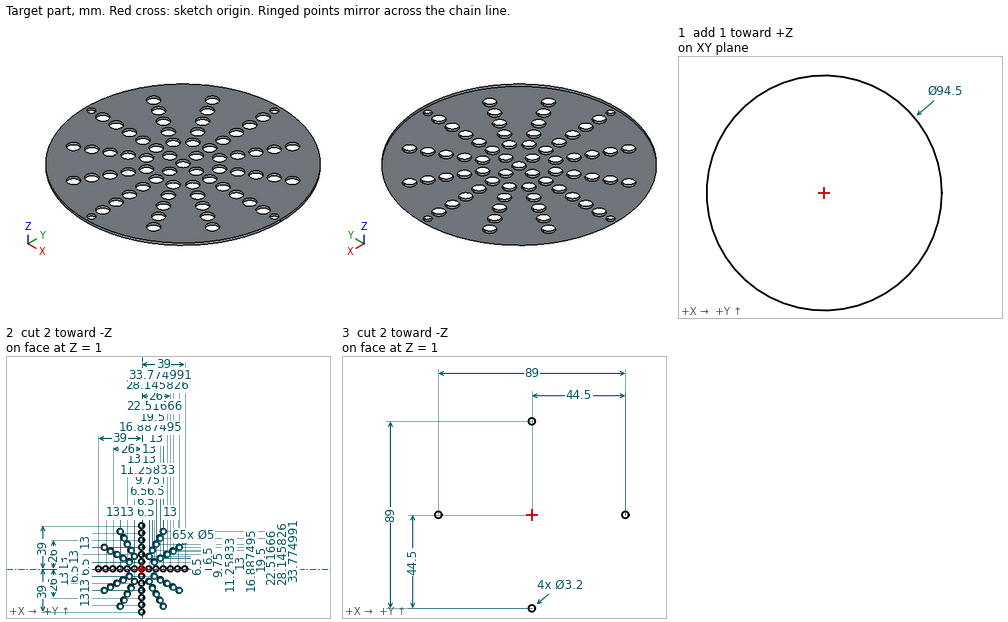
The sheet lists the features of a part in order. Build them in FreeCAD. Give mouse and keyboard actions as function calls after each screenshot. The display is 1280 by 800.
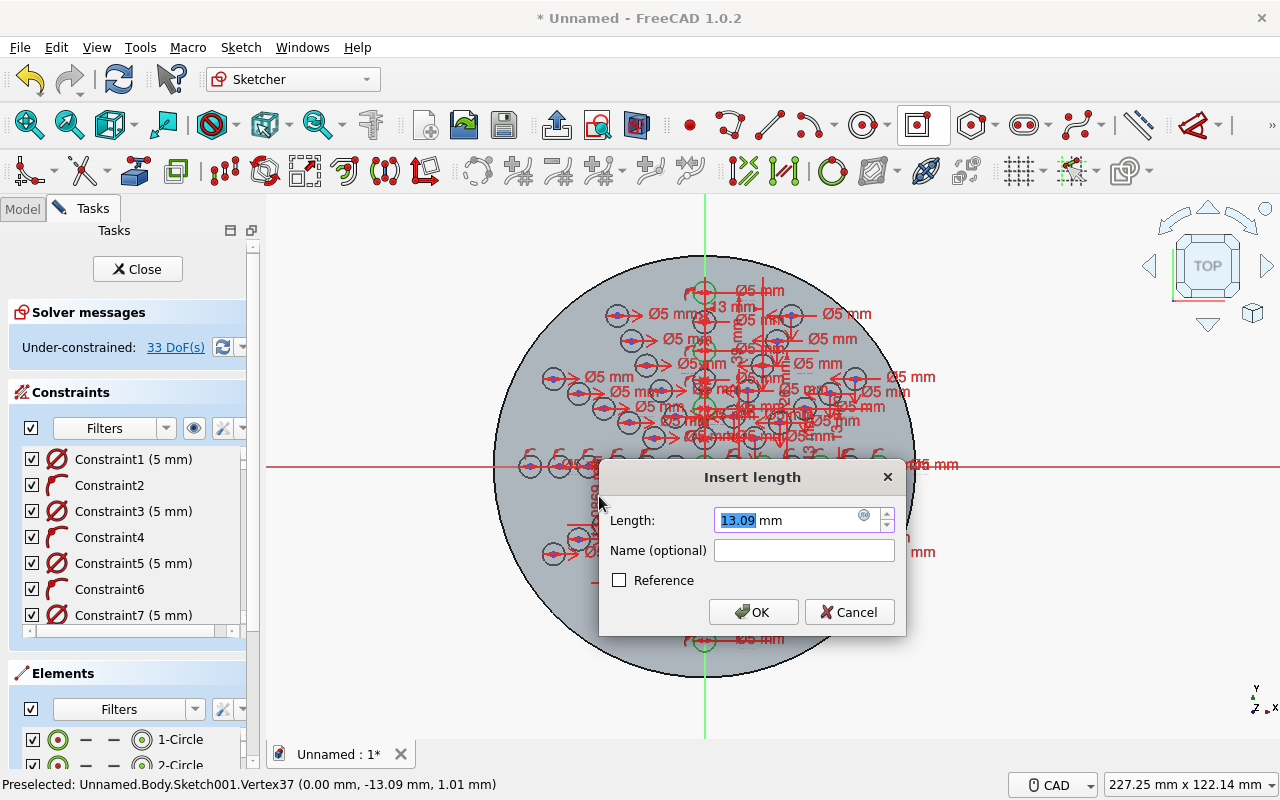
text(13)
key(Return)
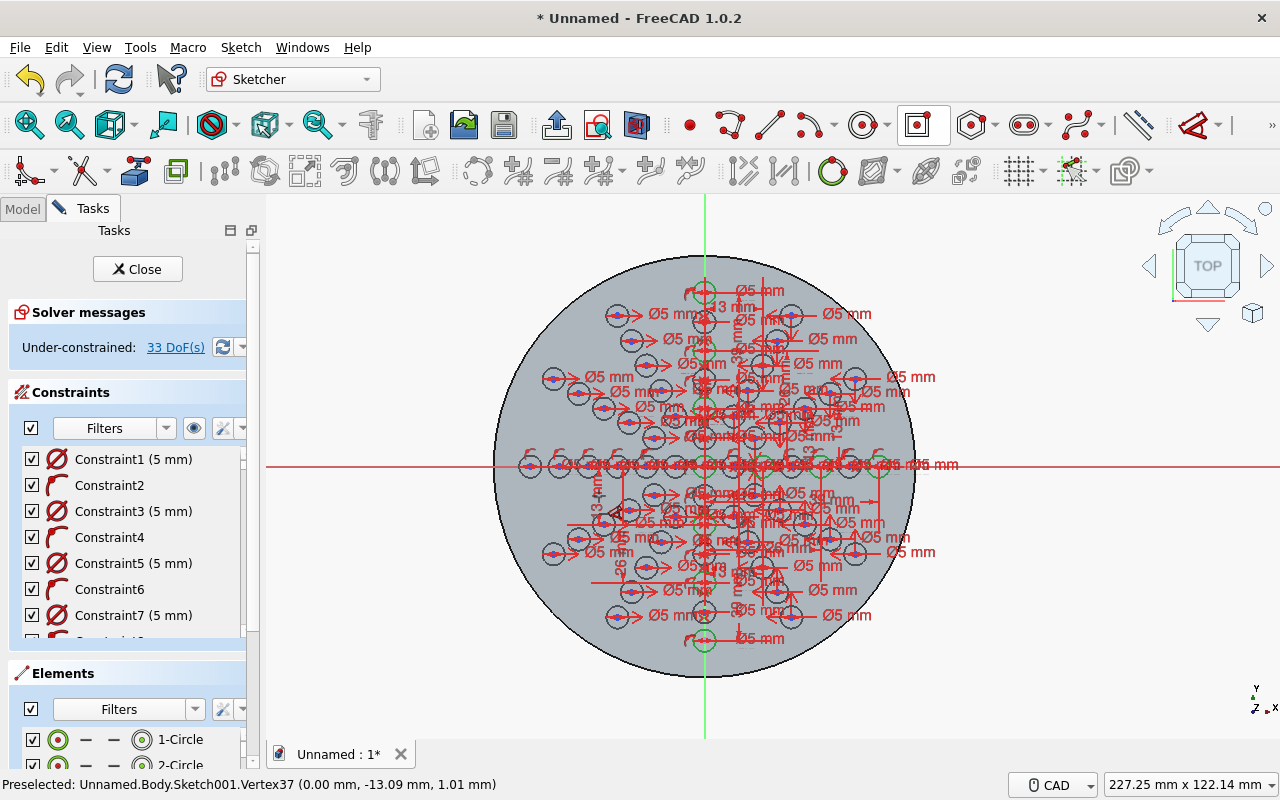
click(530, 467)
click(577, 433)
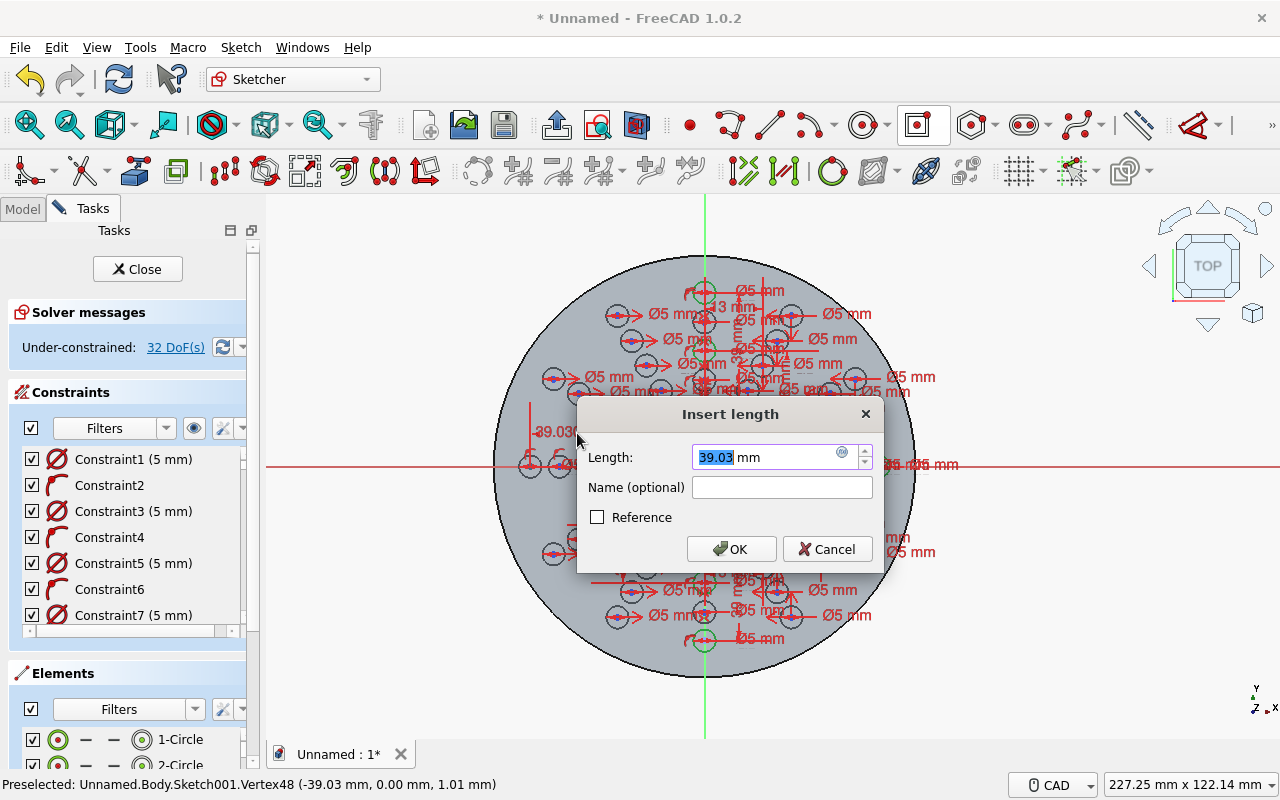
text(39)
key(Return)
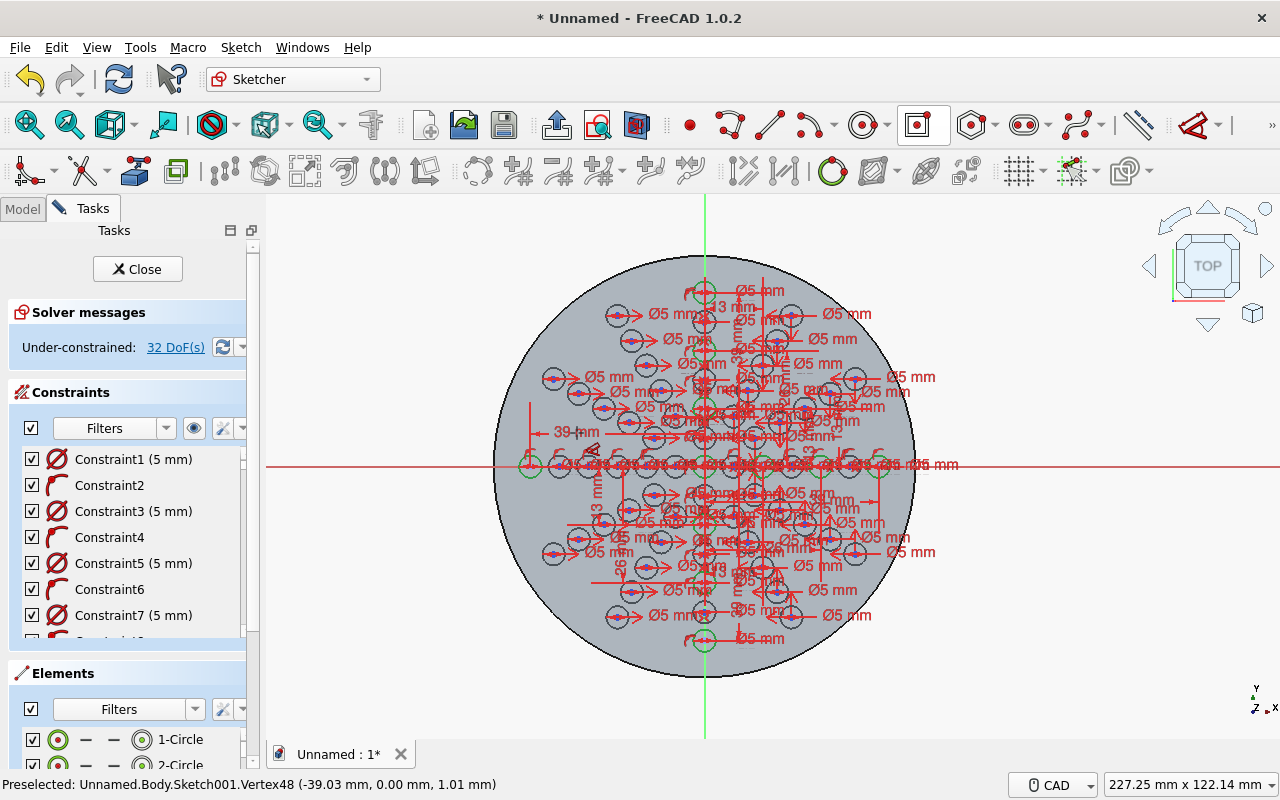
click(588, 467)
click(620, 385)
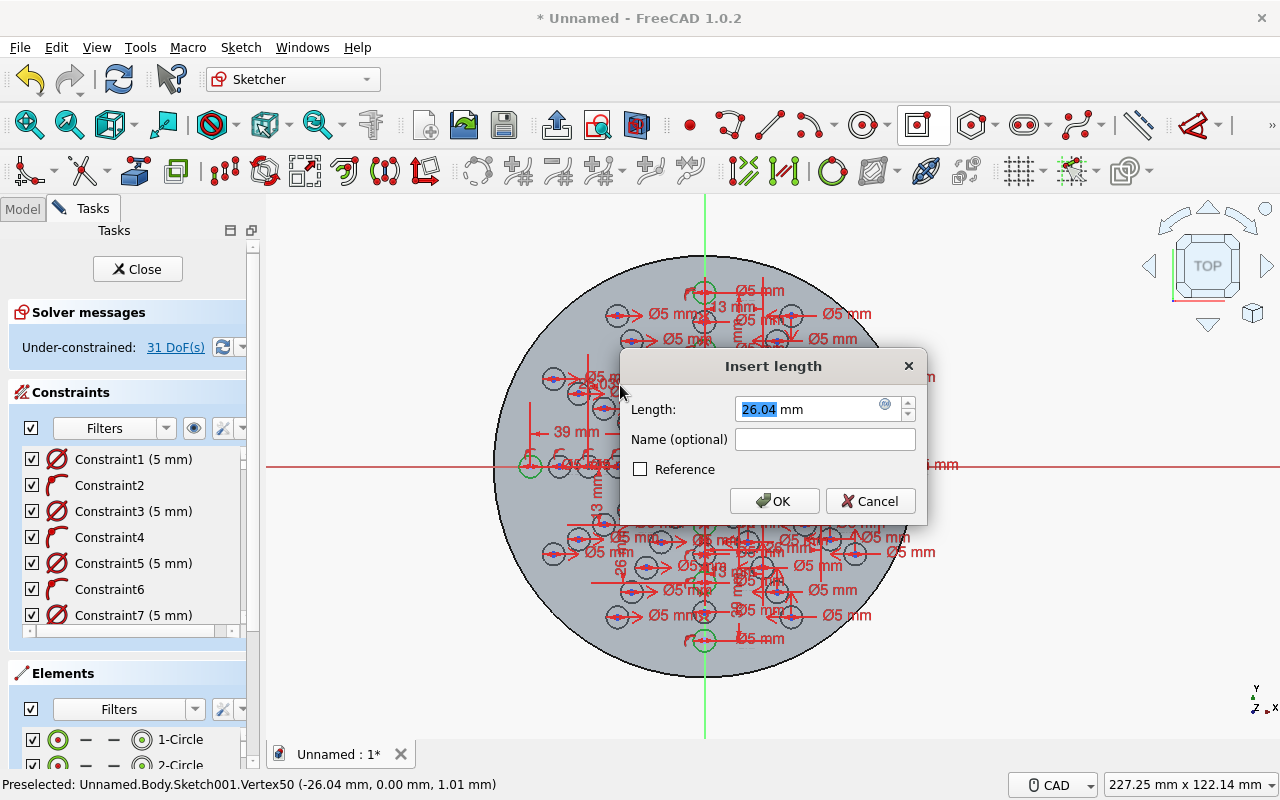
text(26)
key(Return)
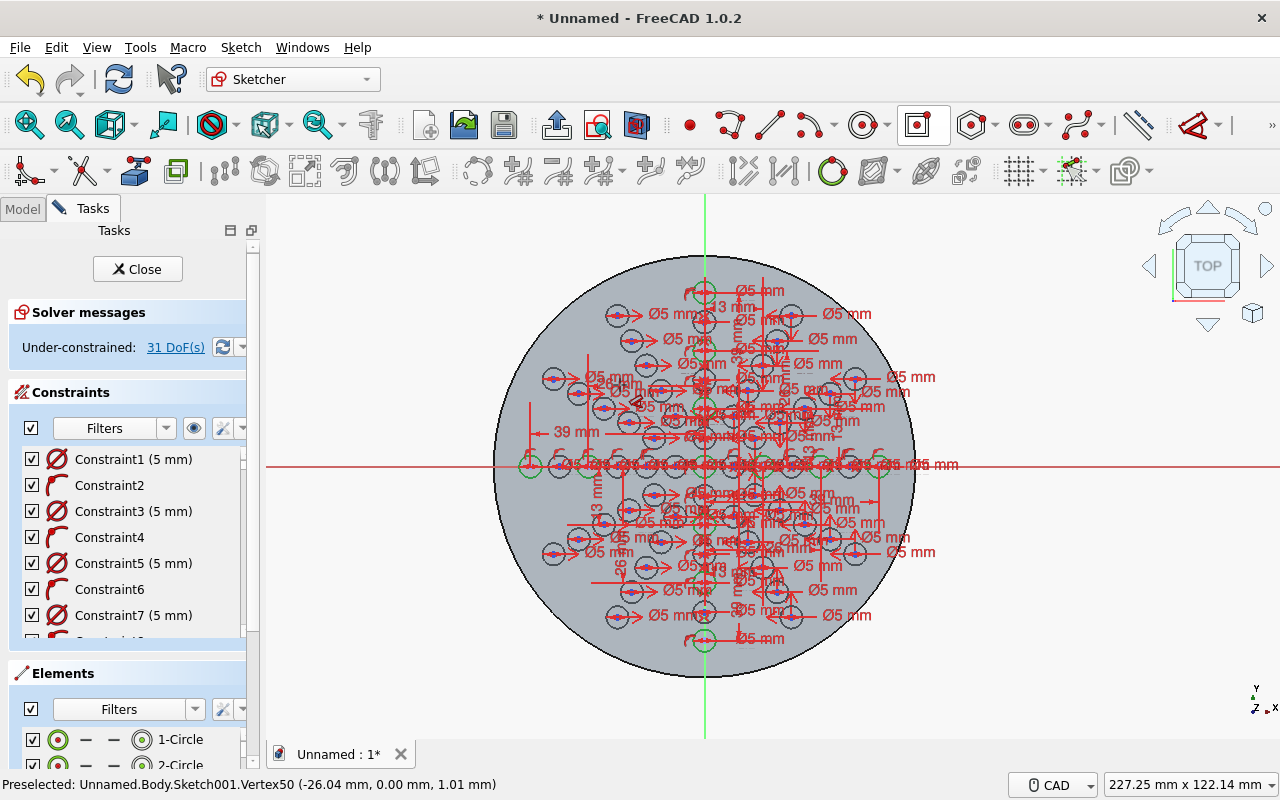
click(646, 467)
click(675, 361)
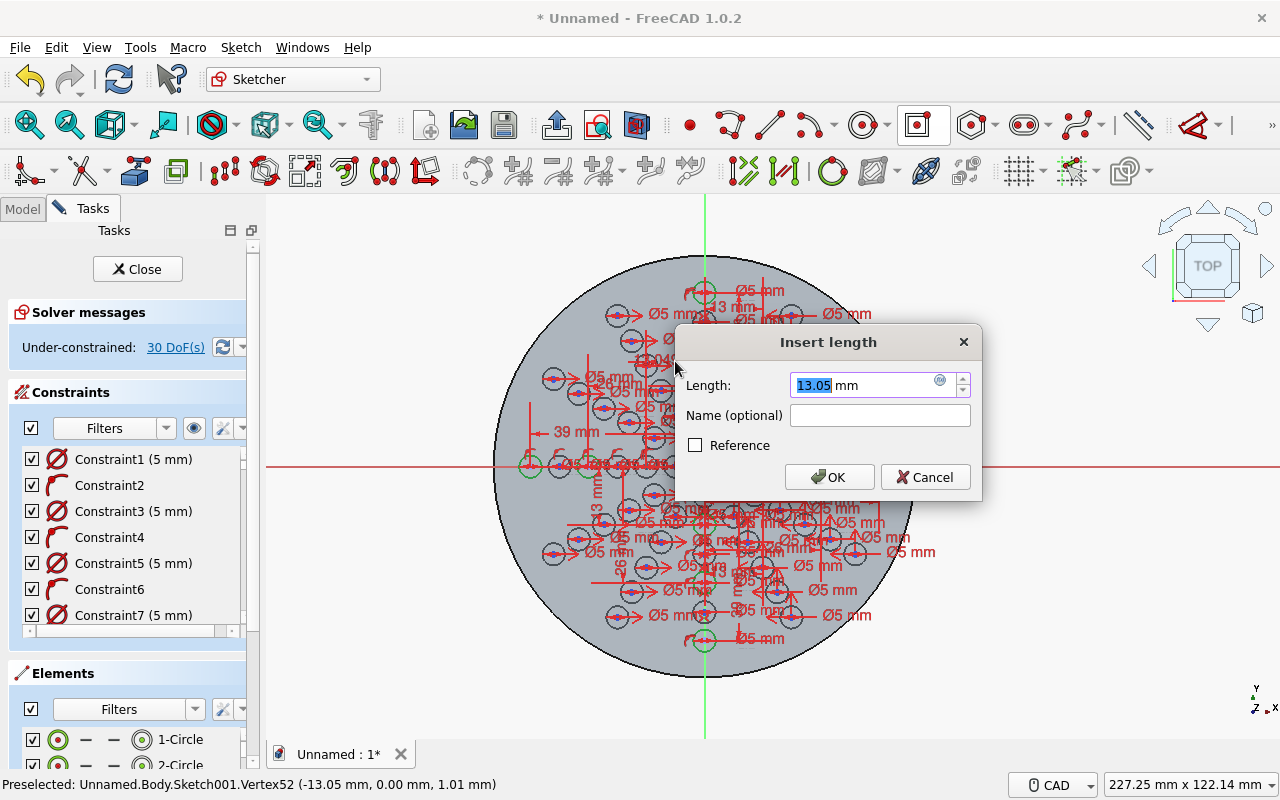
text(13)
key(Return)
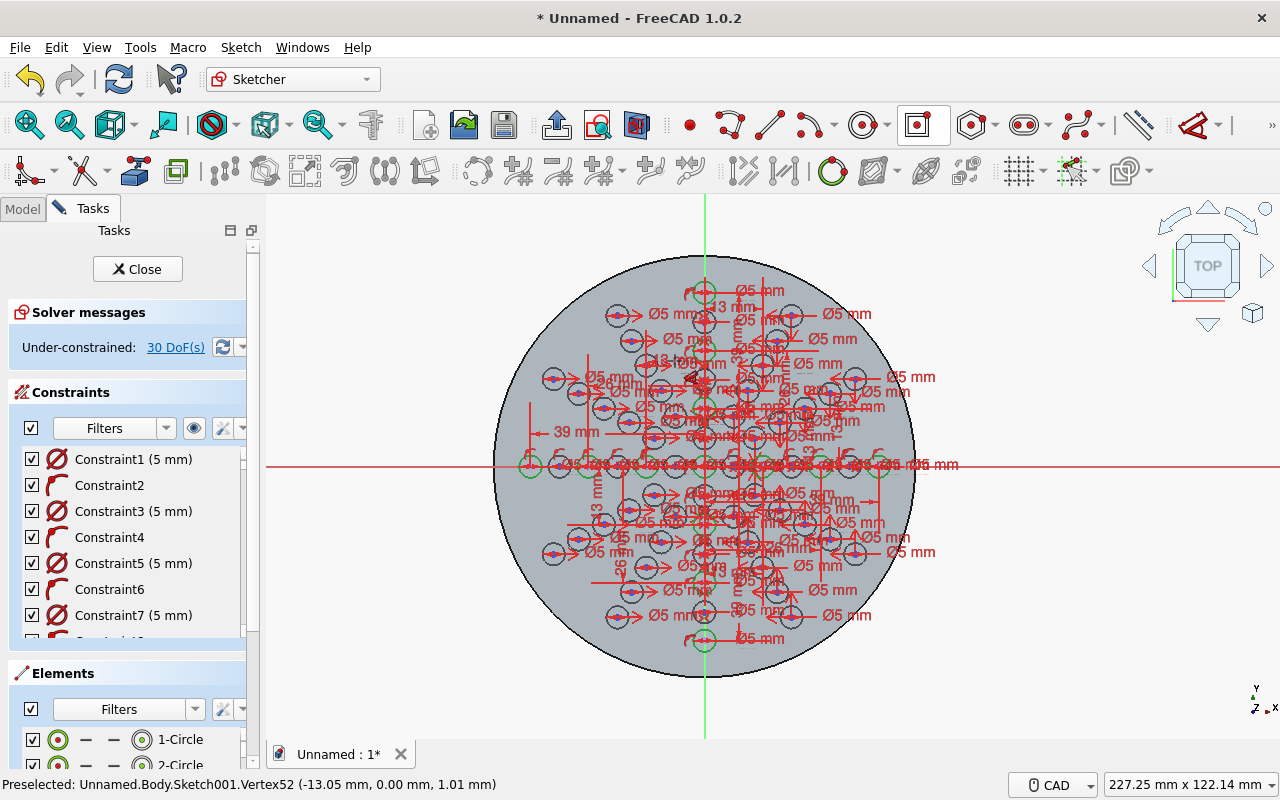
scroll(705, 438, up, 2)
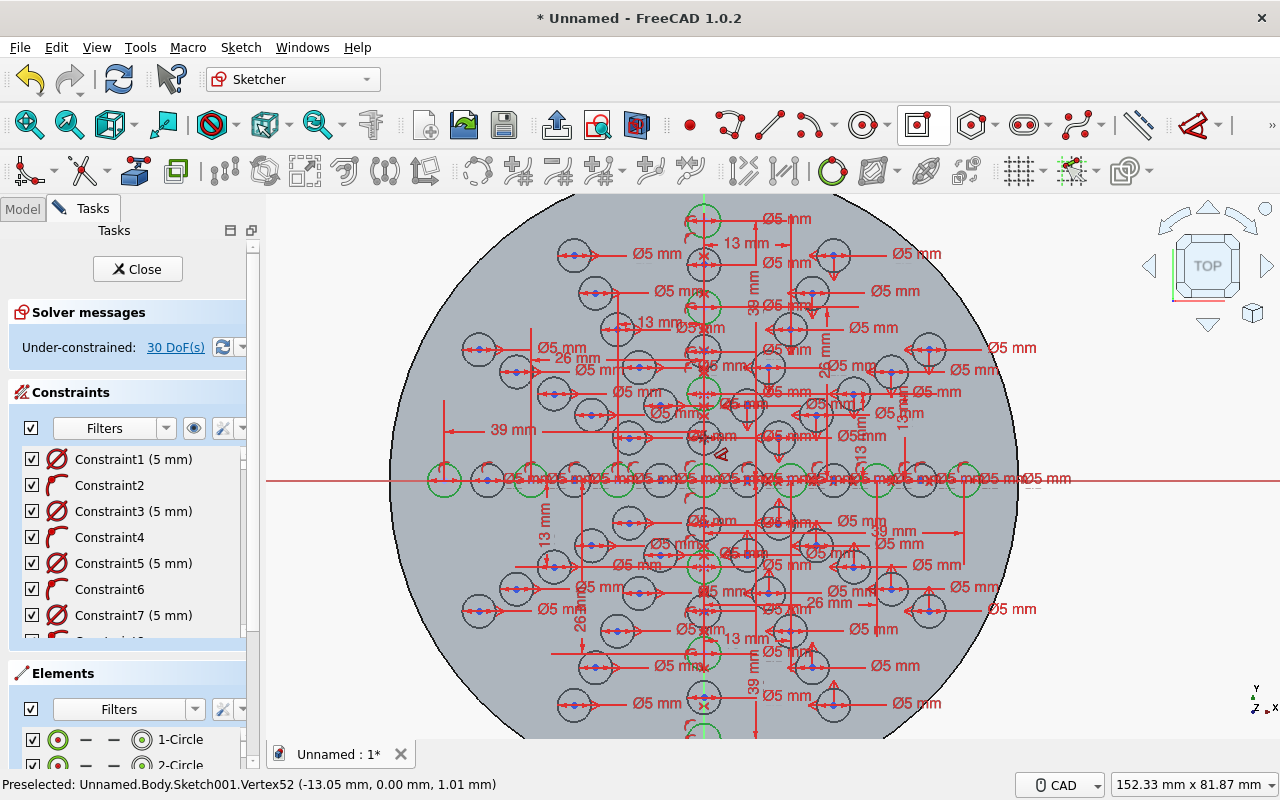
click(704, 438)
click(738, 450)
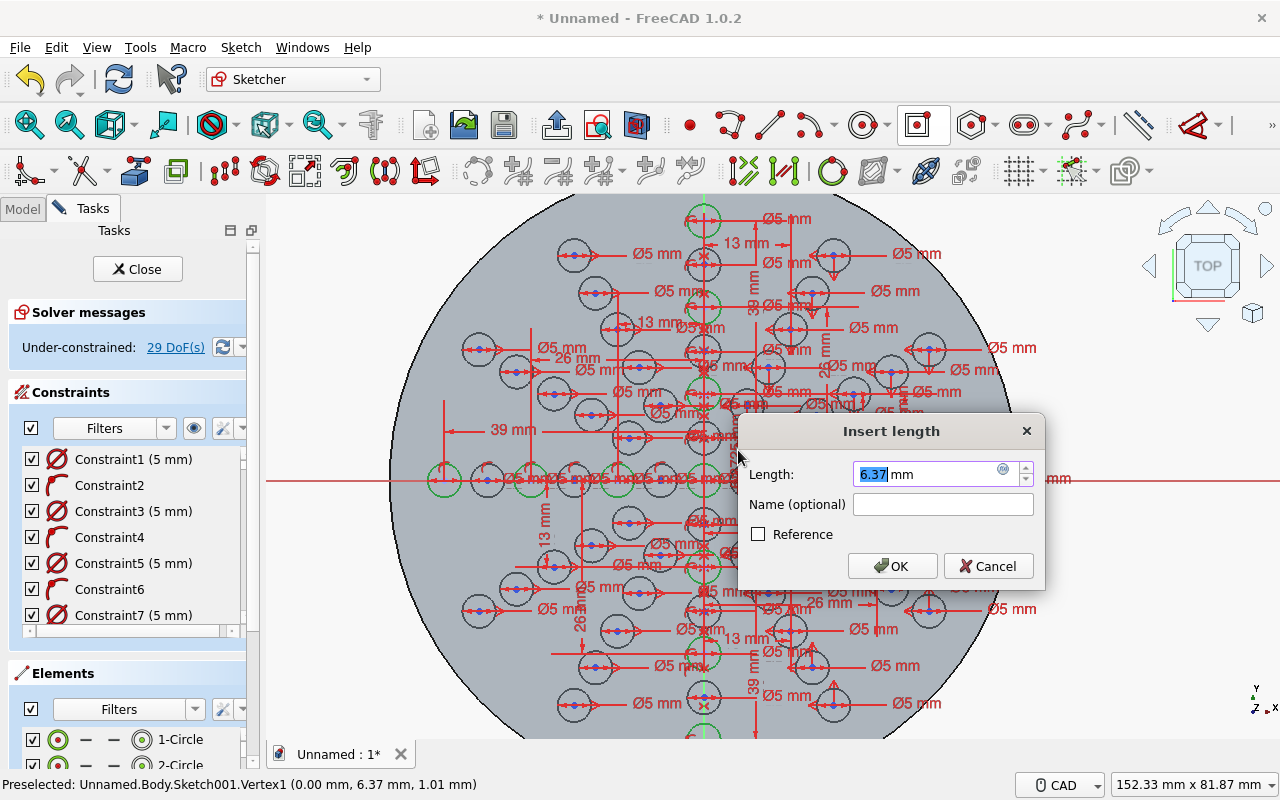
text(6.5)
key(Return)